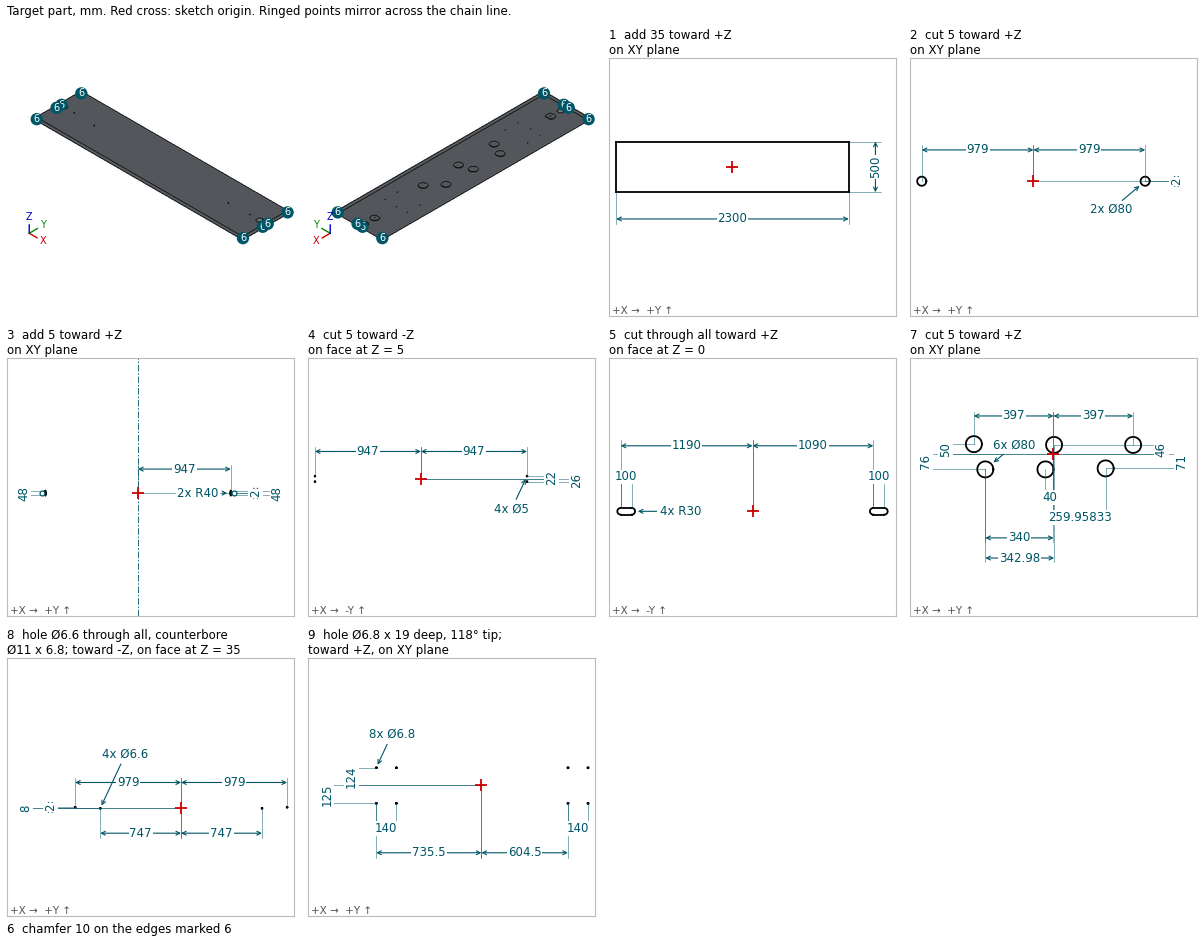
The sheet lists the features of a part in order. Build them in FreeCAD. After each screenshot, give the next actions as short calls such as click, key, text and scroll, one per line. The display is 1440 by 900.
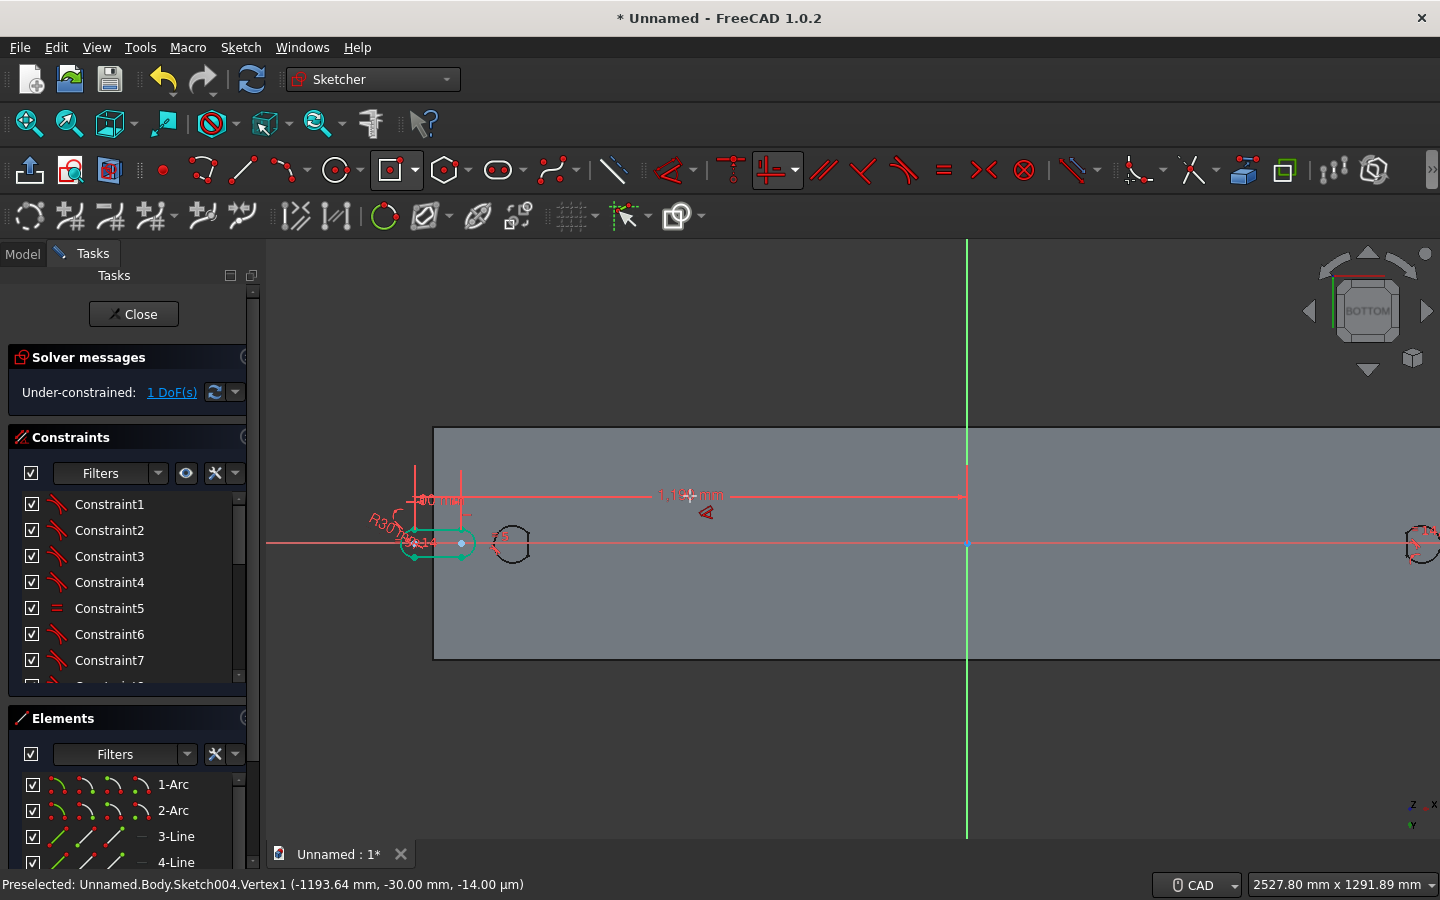
scroll(413, 530, down, 2)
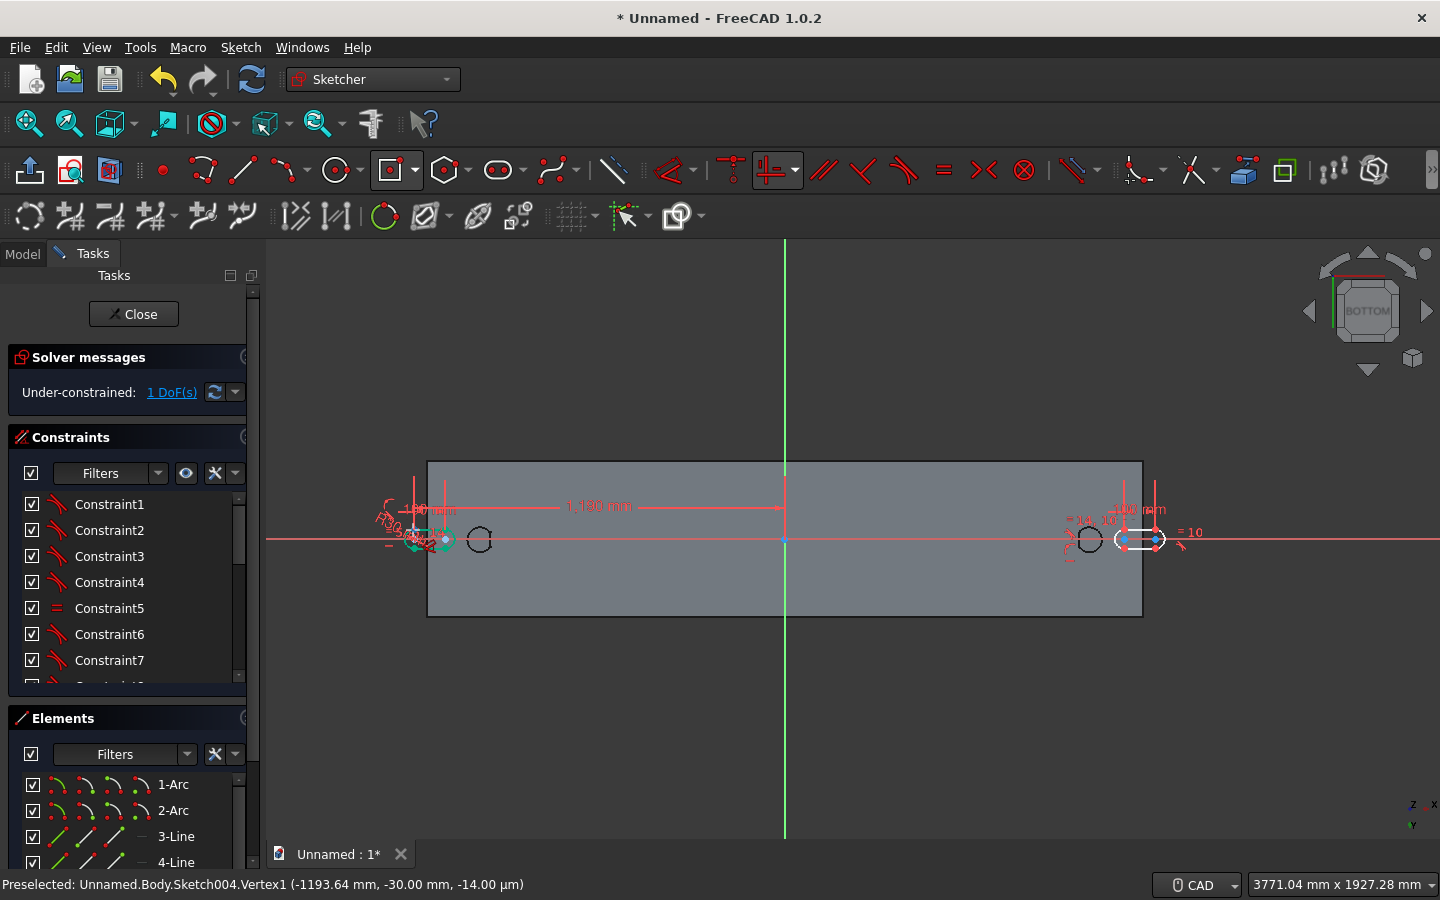
scroll(1124, 530, up, 2)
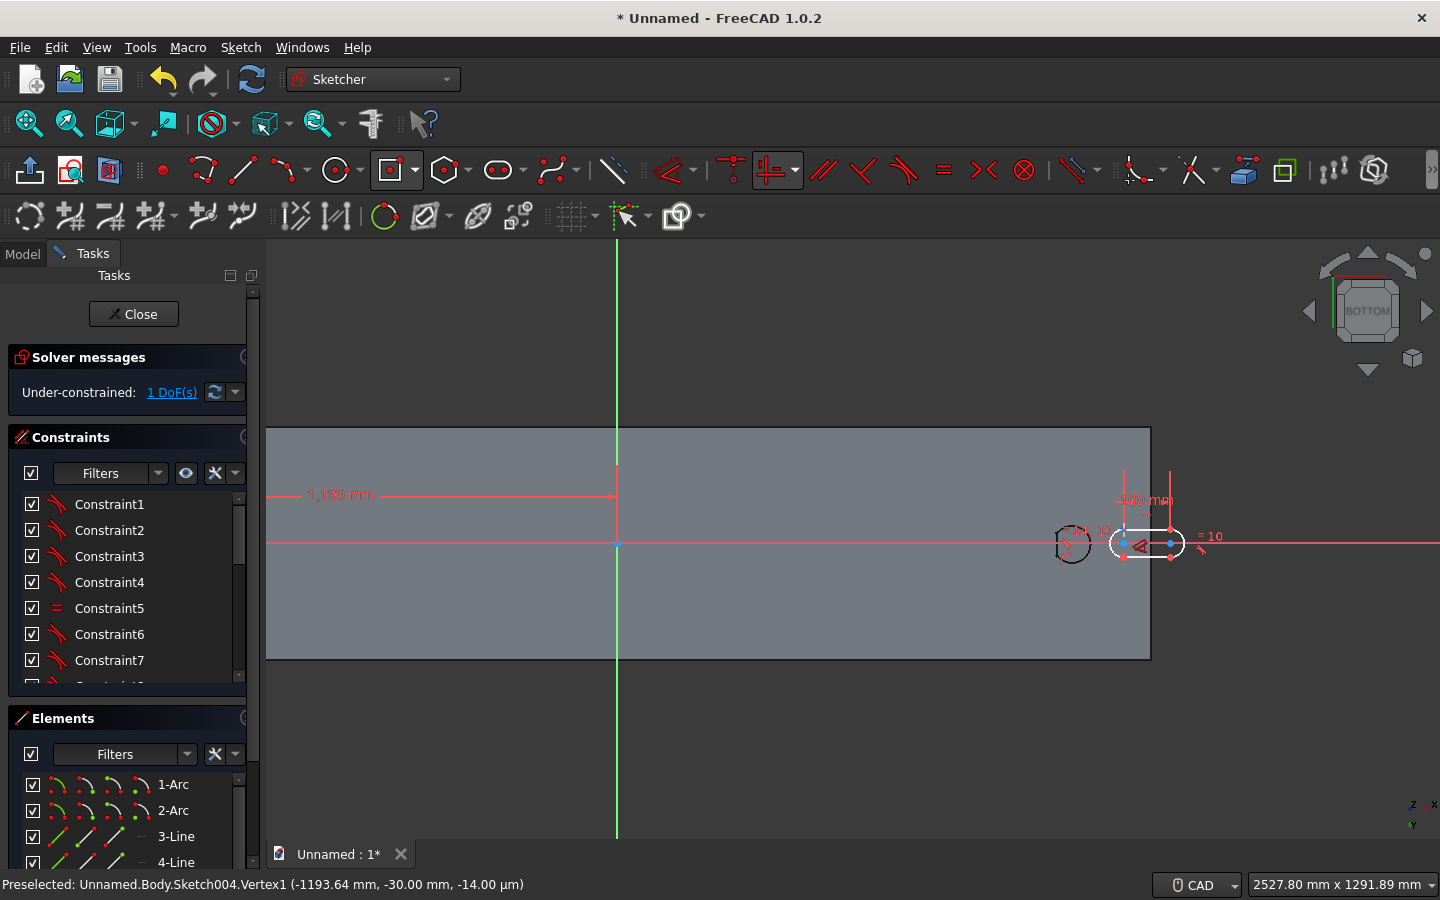
click(1124, 530)
click(871, 496)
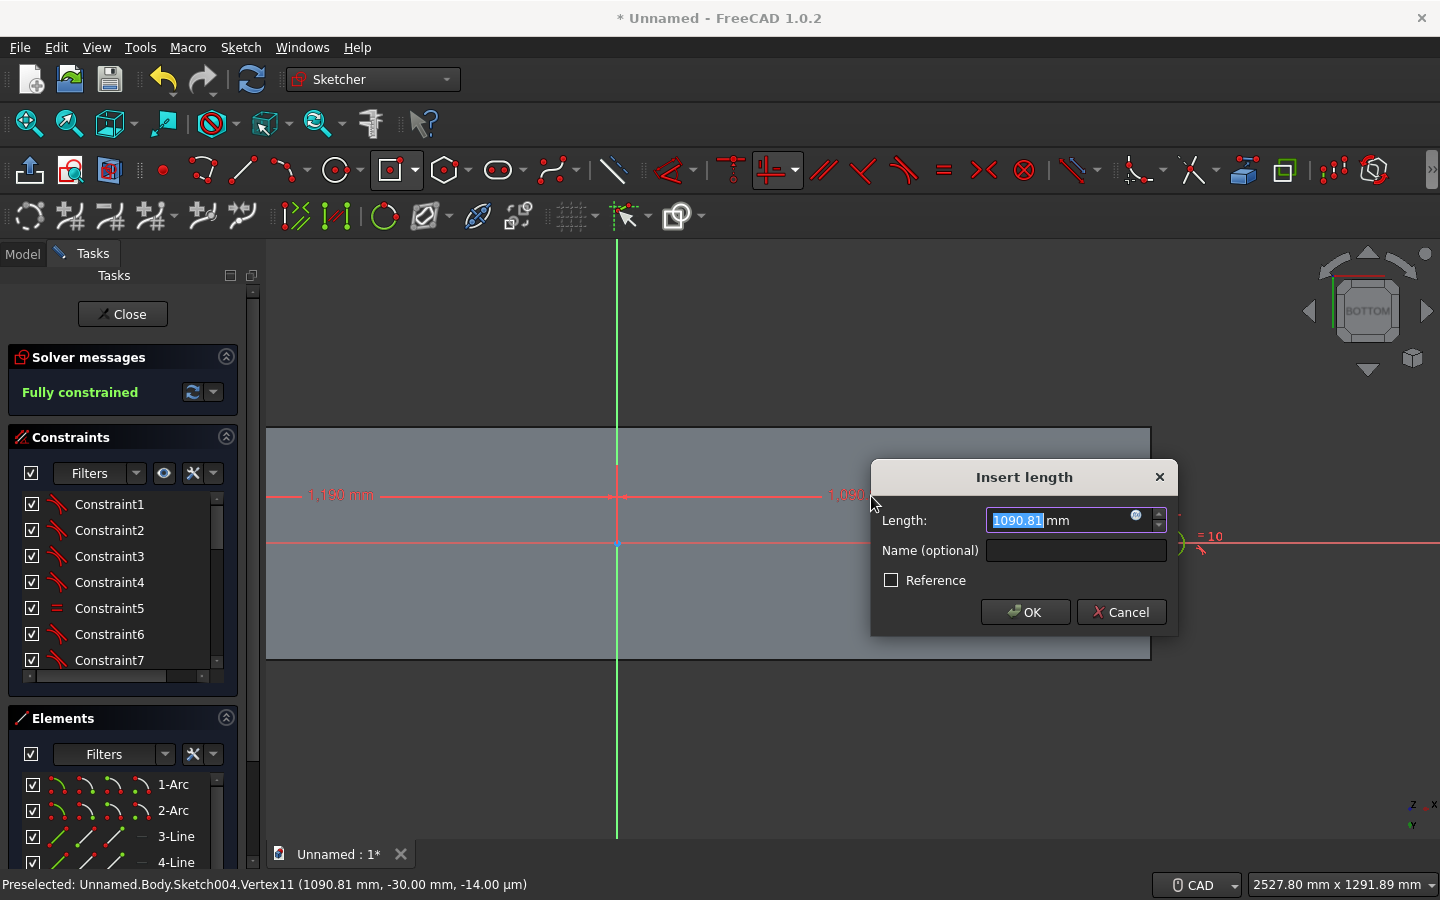
text(1090)
key(Return)
key(Escape)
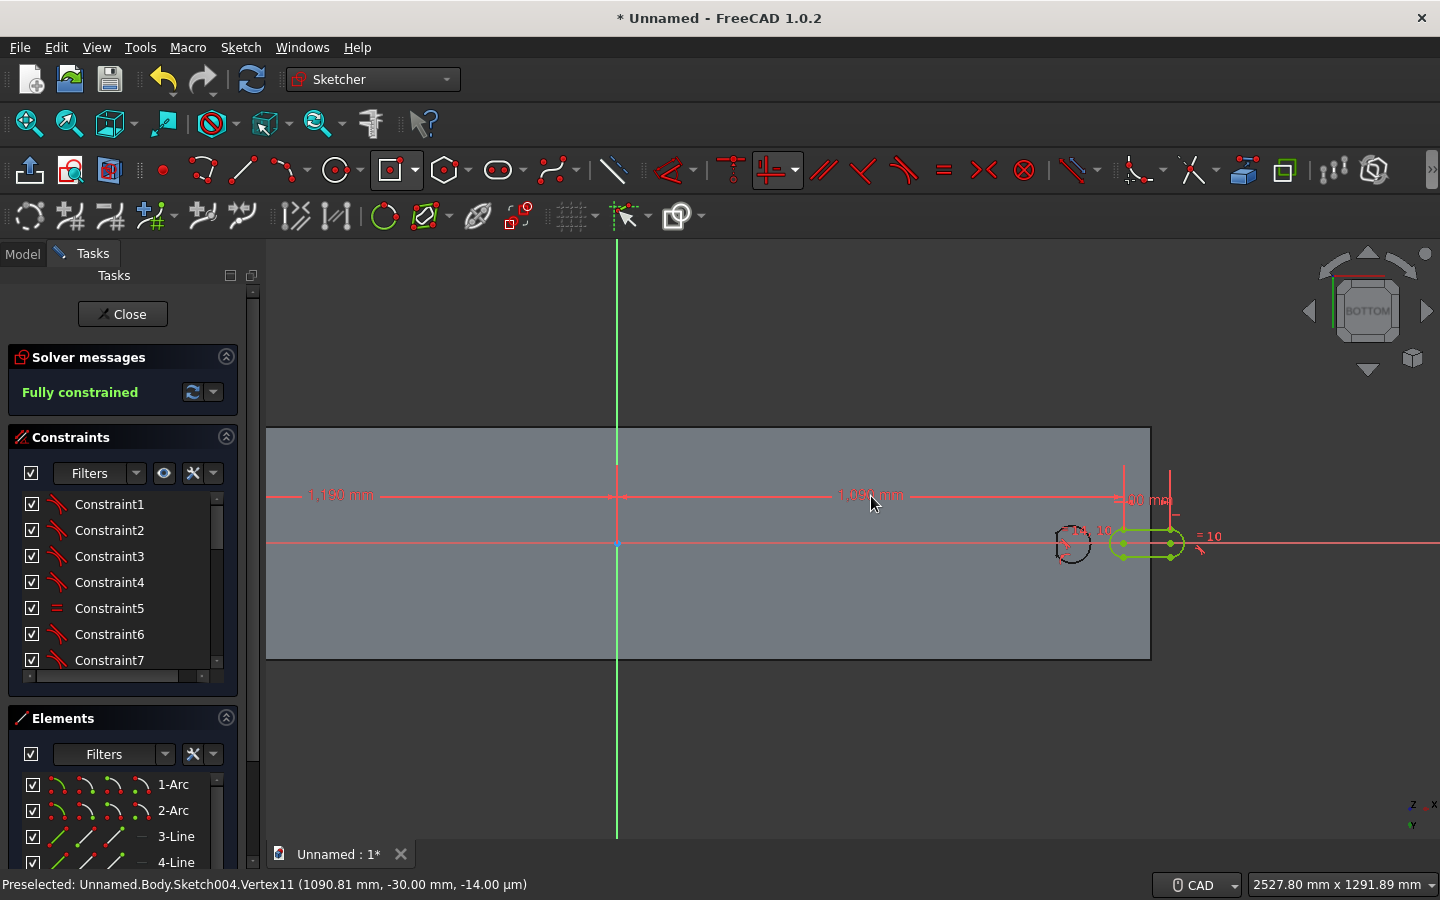
click(123, 314)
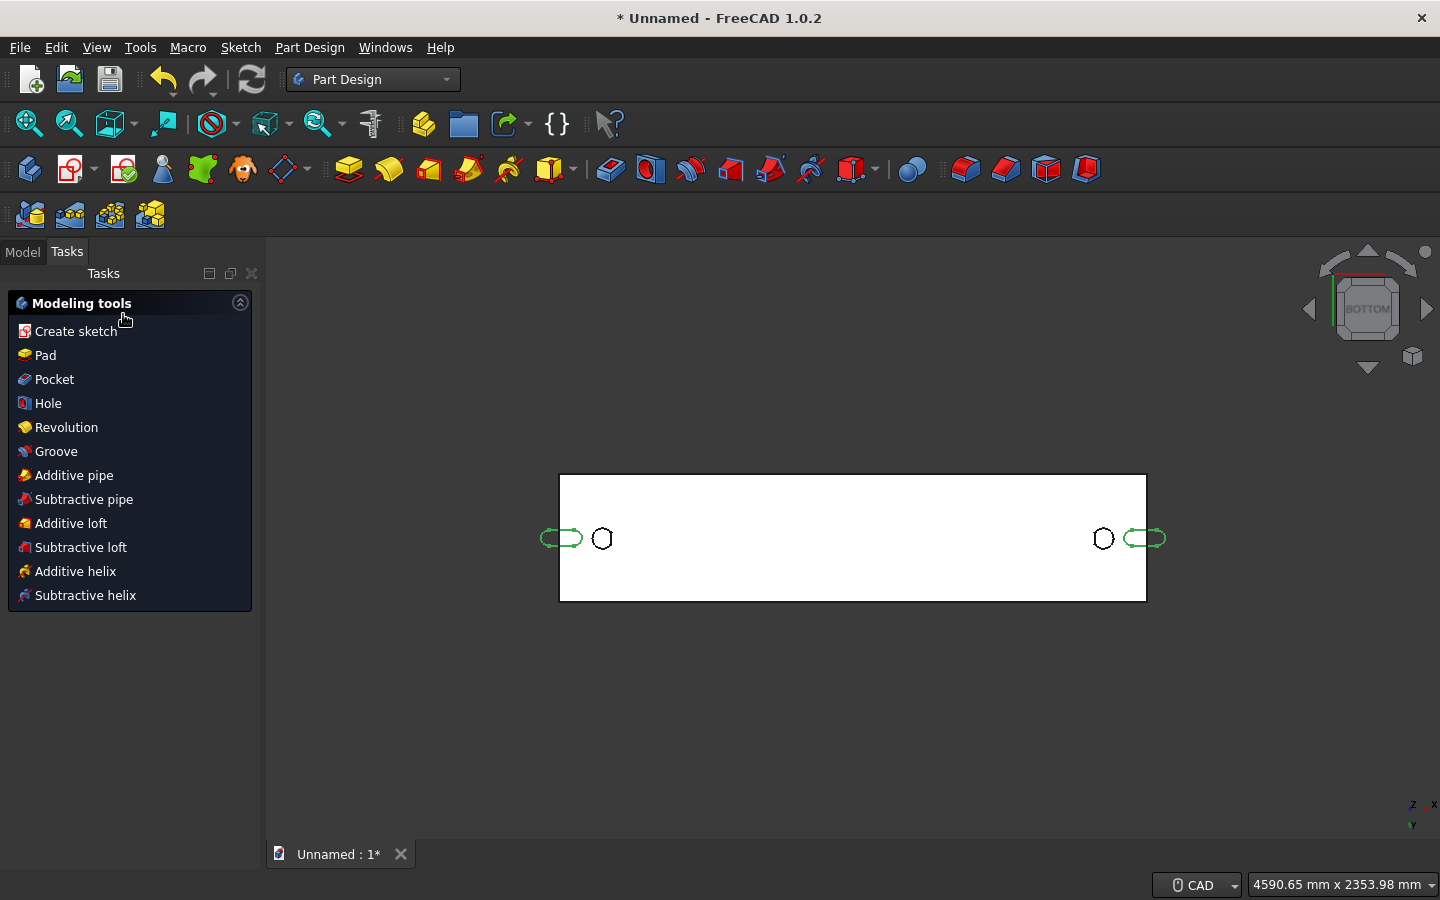
click(612, 170)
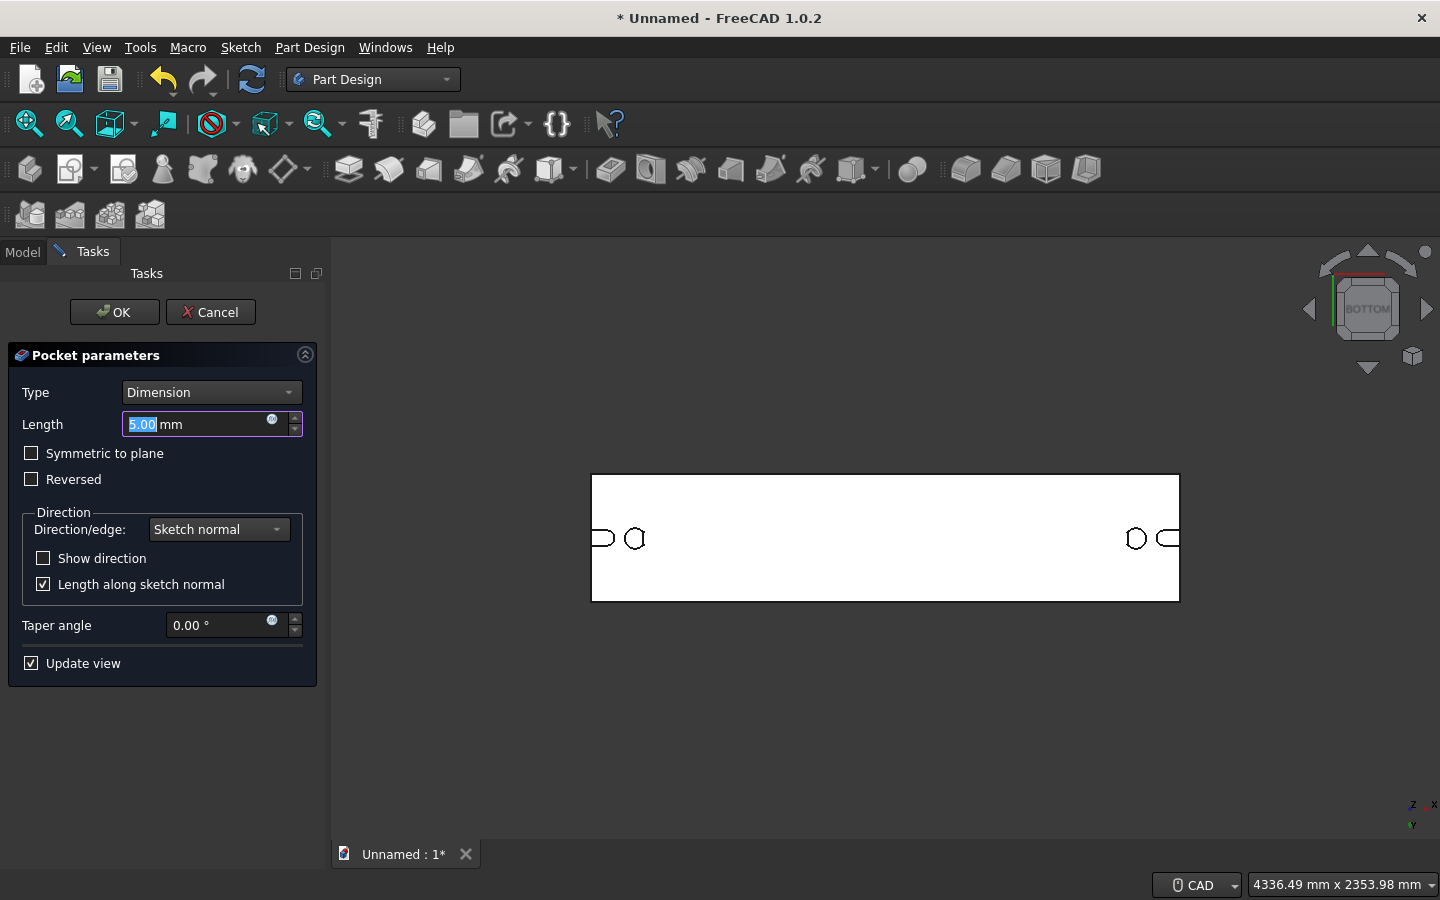
click(212, 392)